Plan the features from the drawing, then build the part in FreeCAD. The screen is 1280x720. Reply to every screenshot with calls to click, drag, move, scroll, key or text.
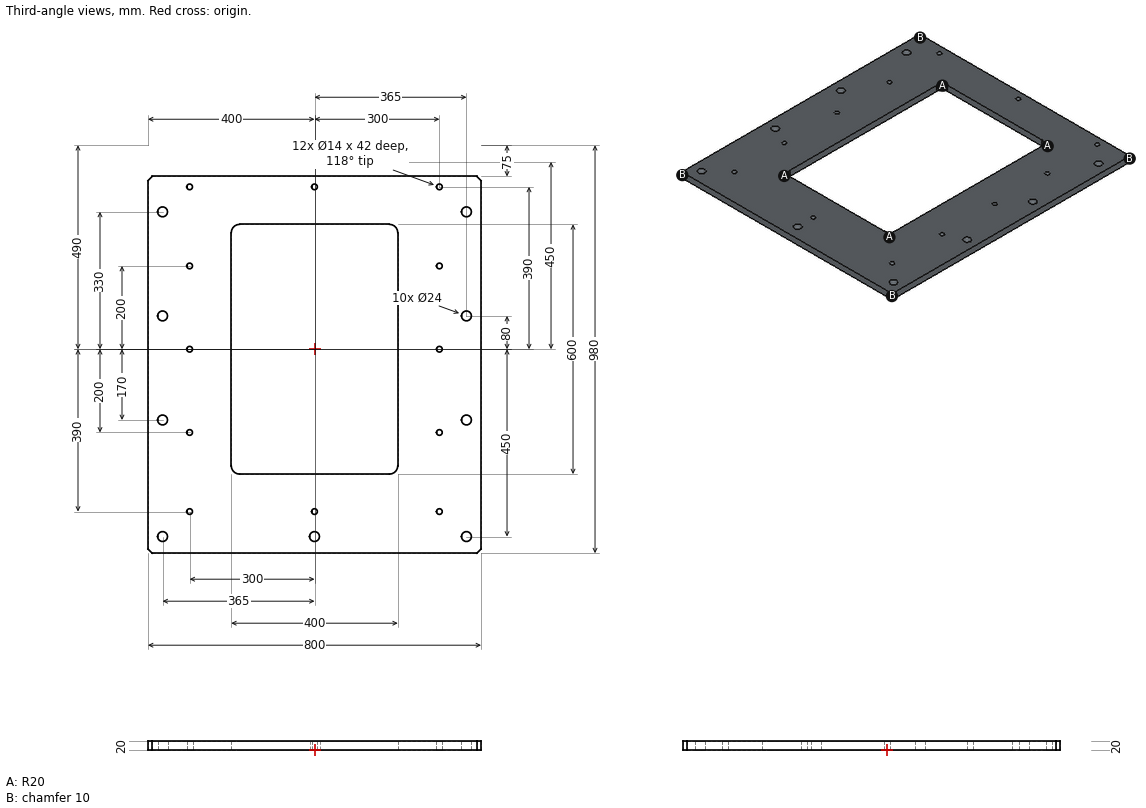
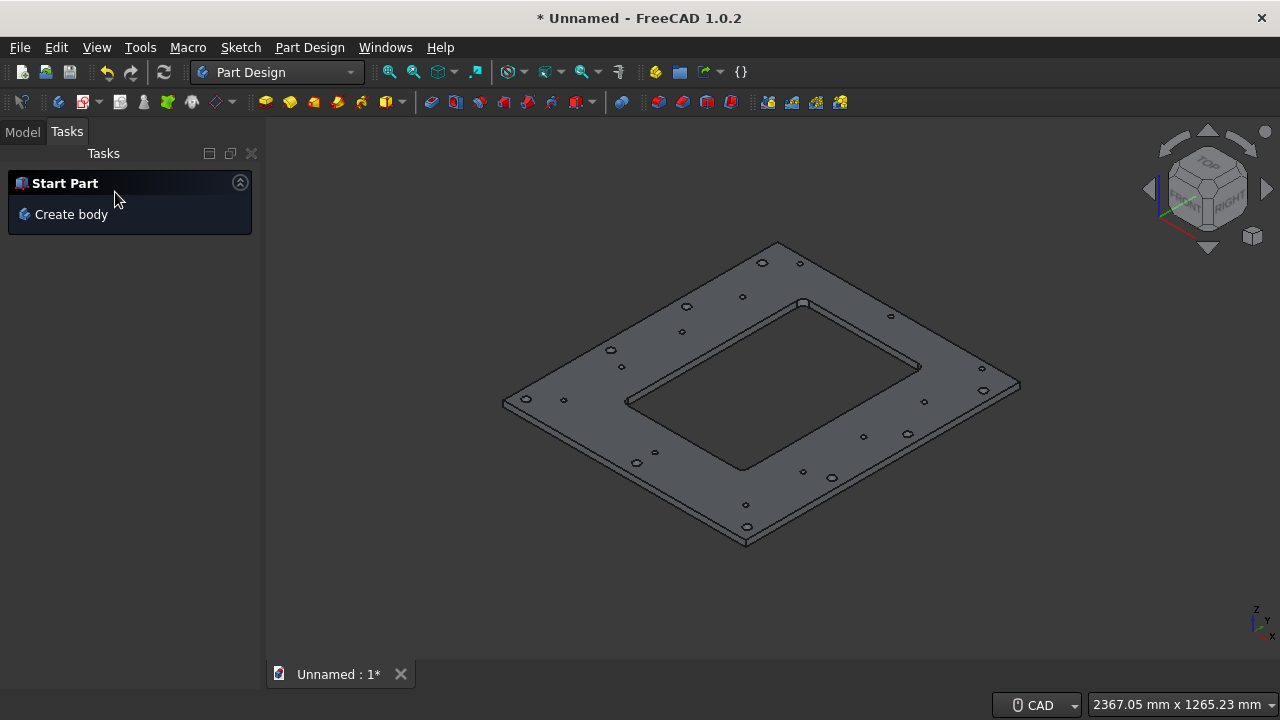
scroll(778, 244, up, 8)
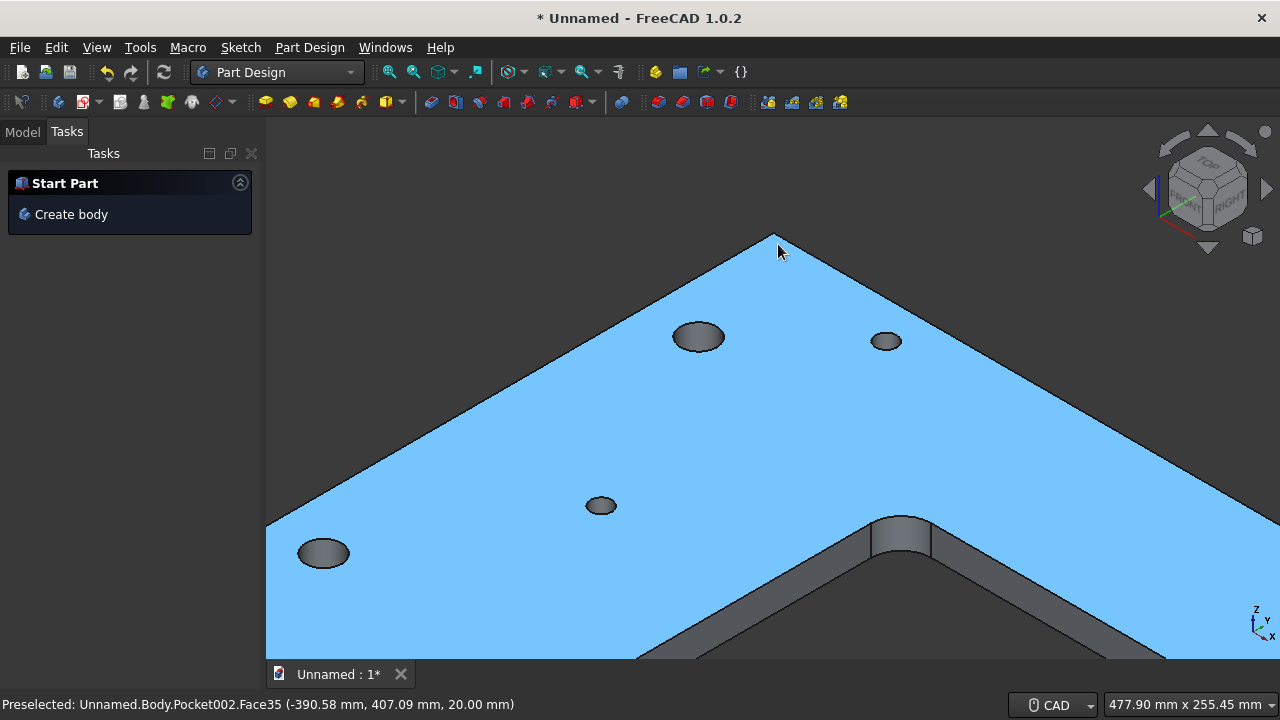
click(390, 72)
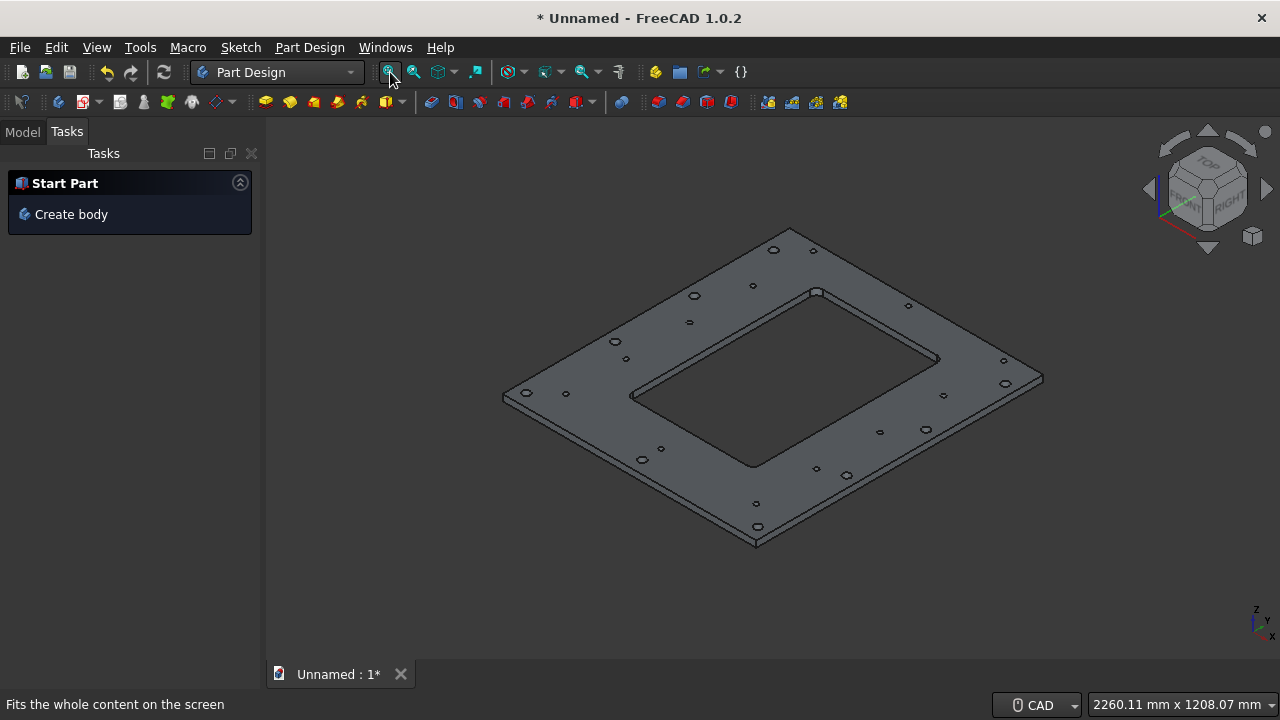
key(2)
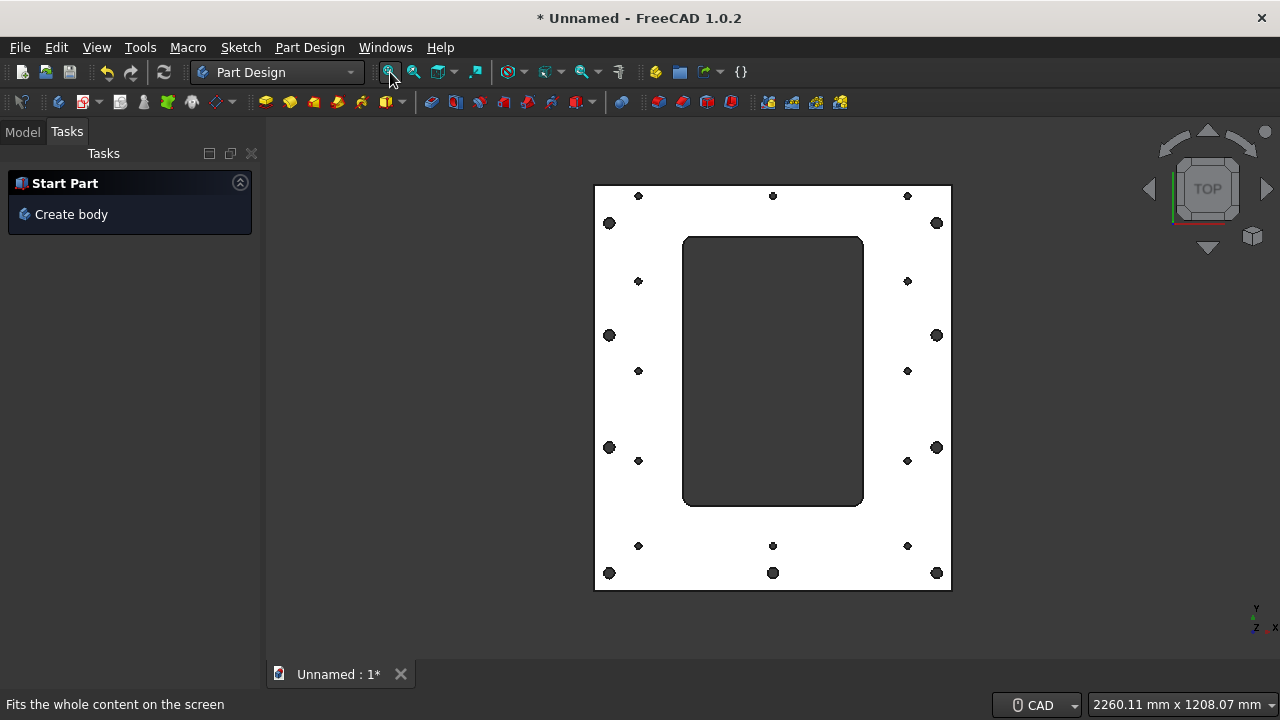
scroll(594, 184, up, 8)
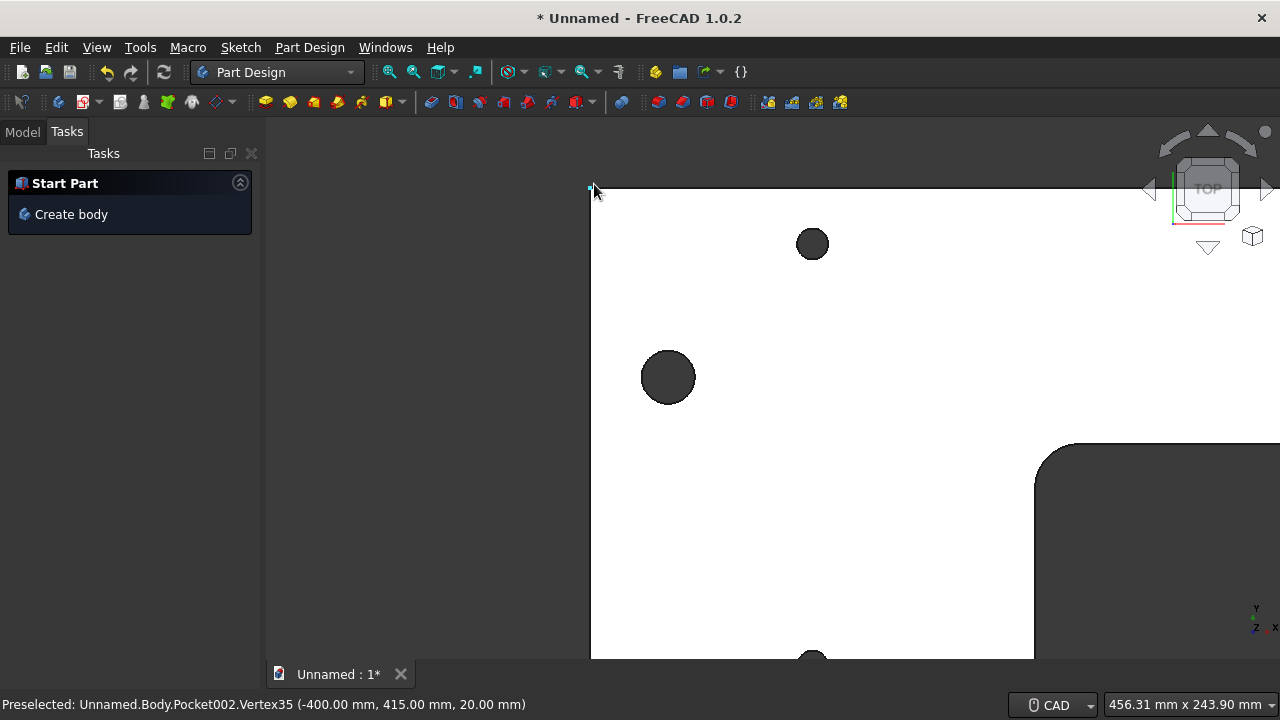
click(390, 72)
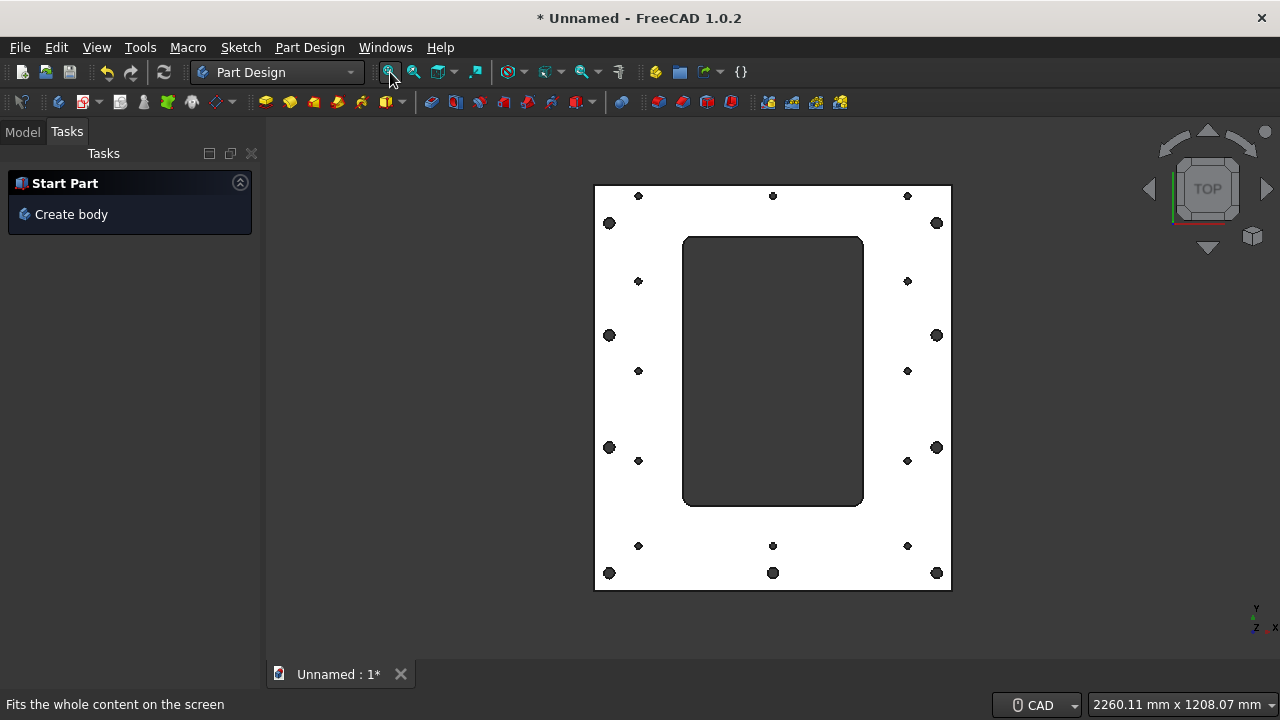
key(0)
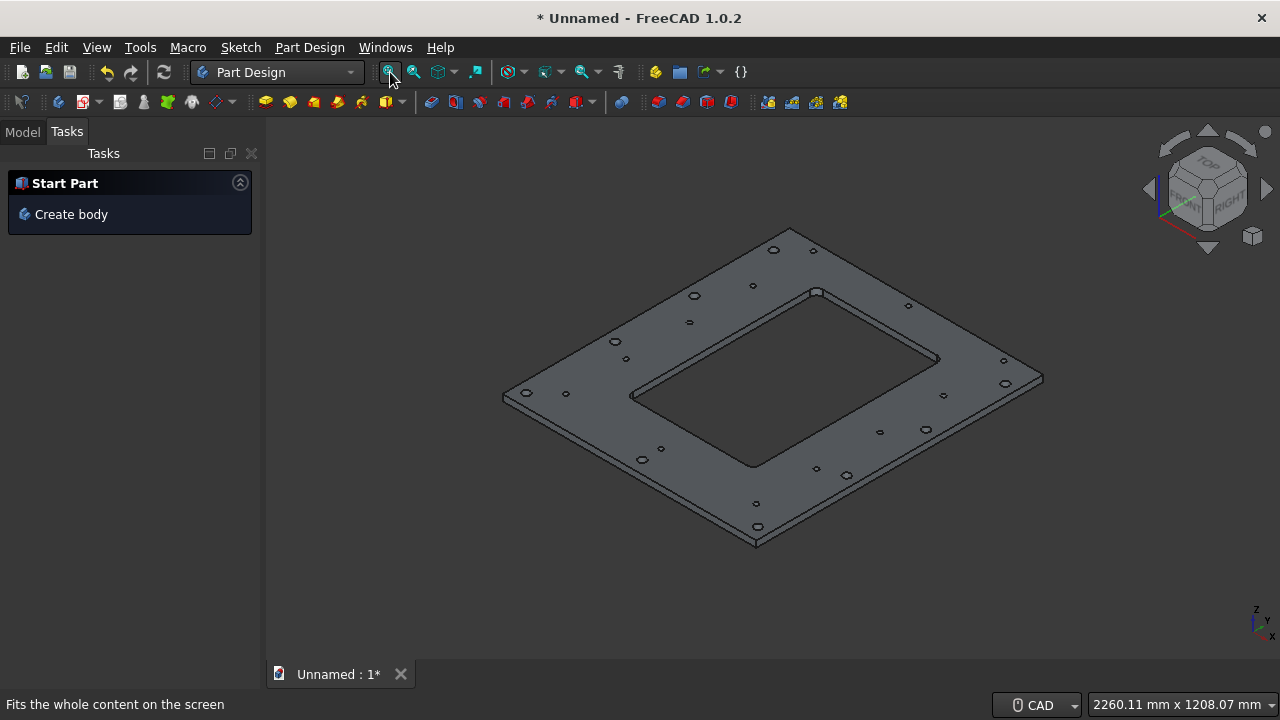
scroll(790, 231, up, 8)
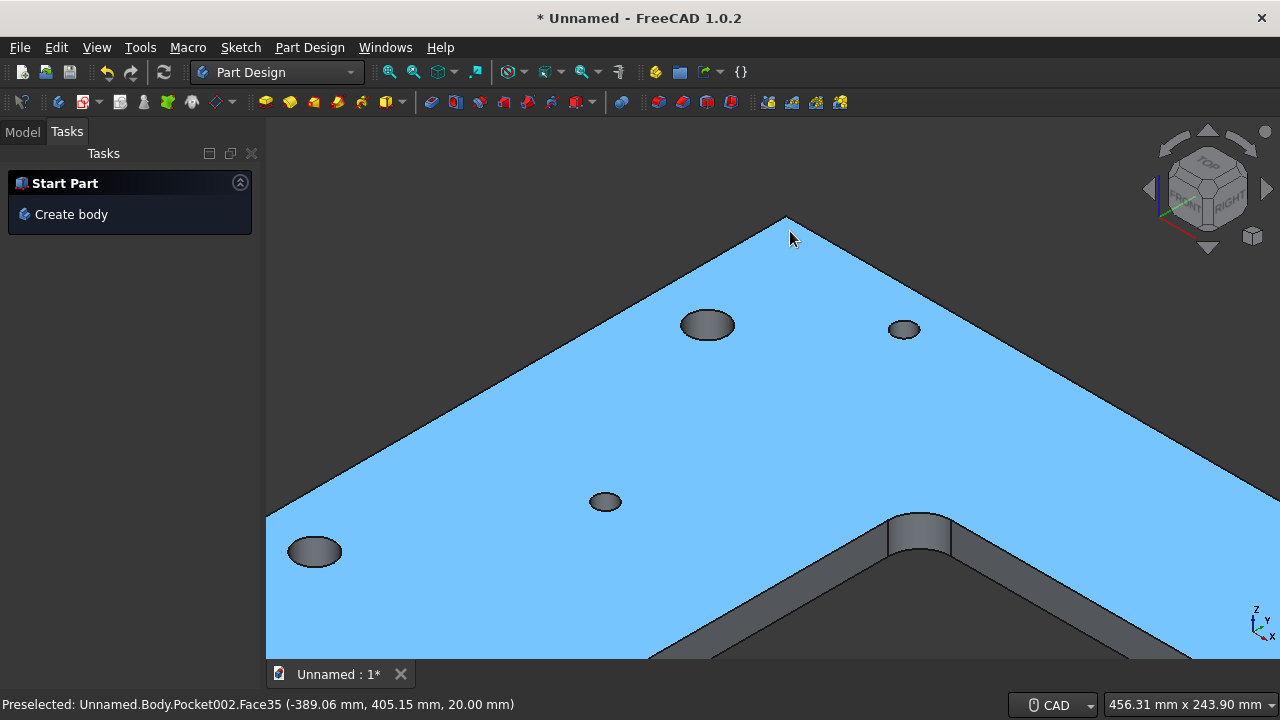
click(390, 72)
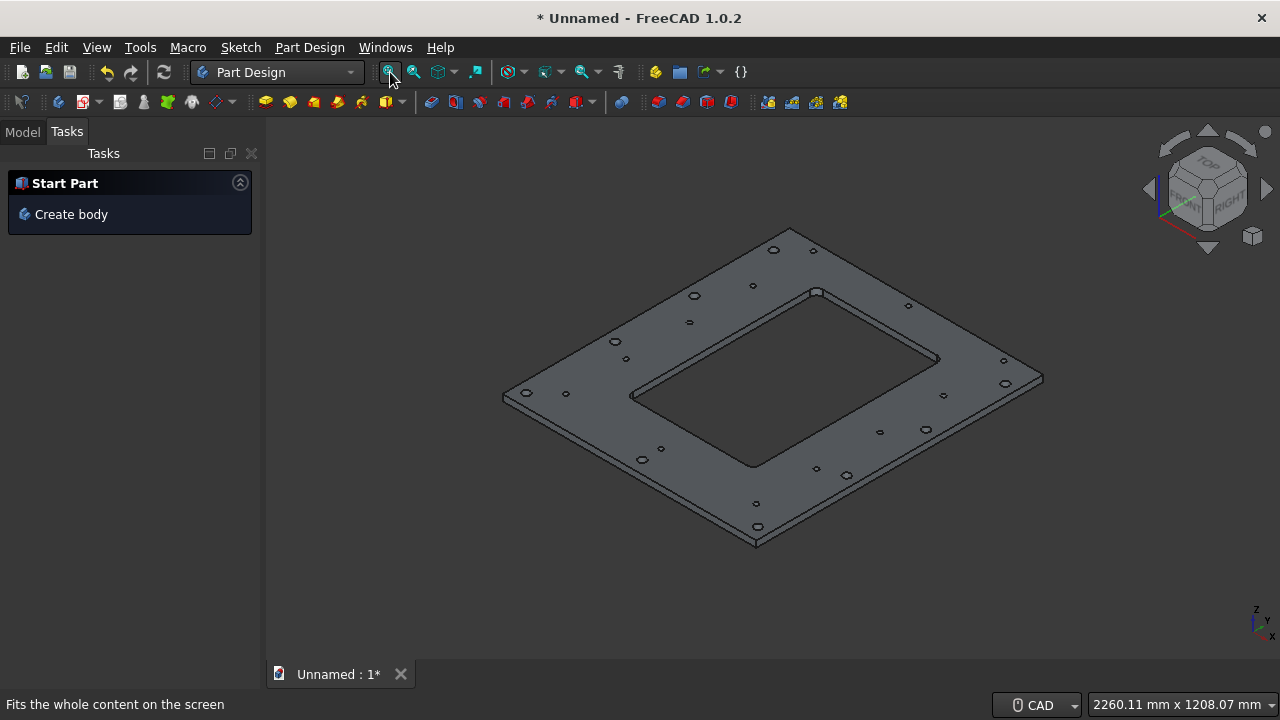
key(1)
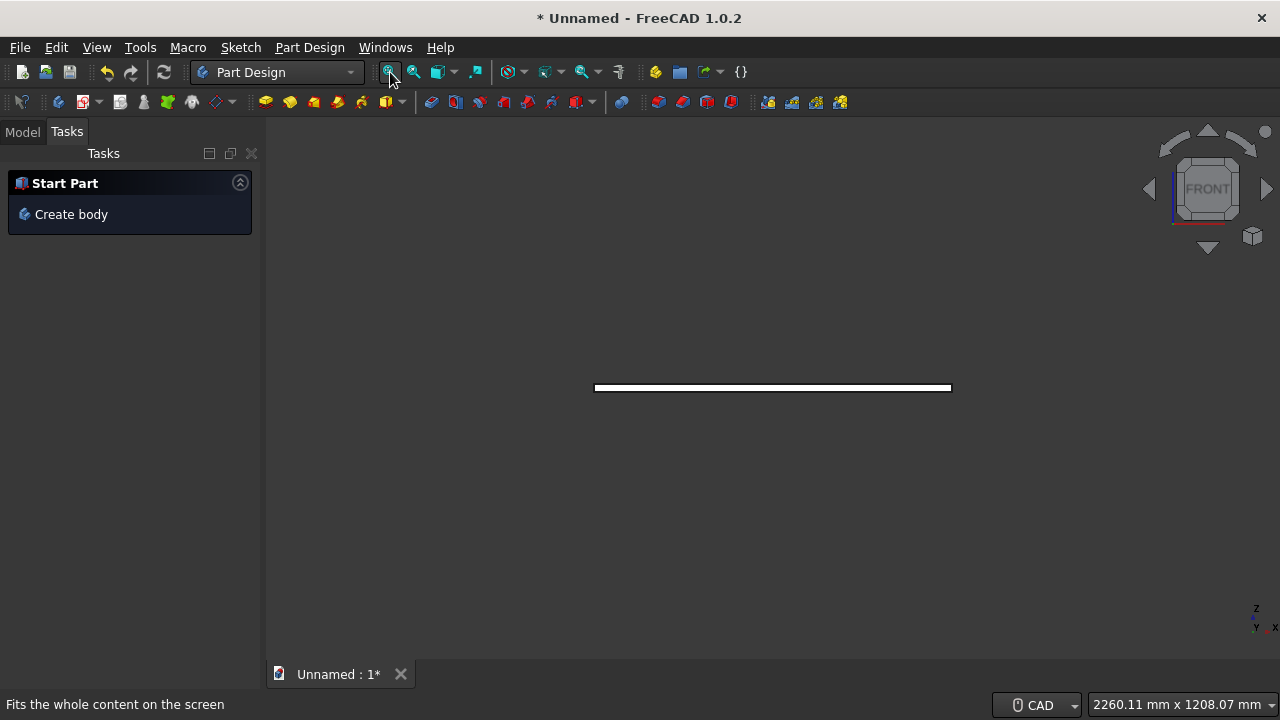
click(390, 72)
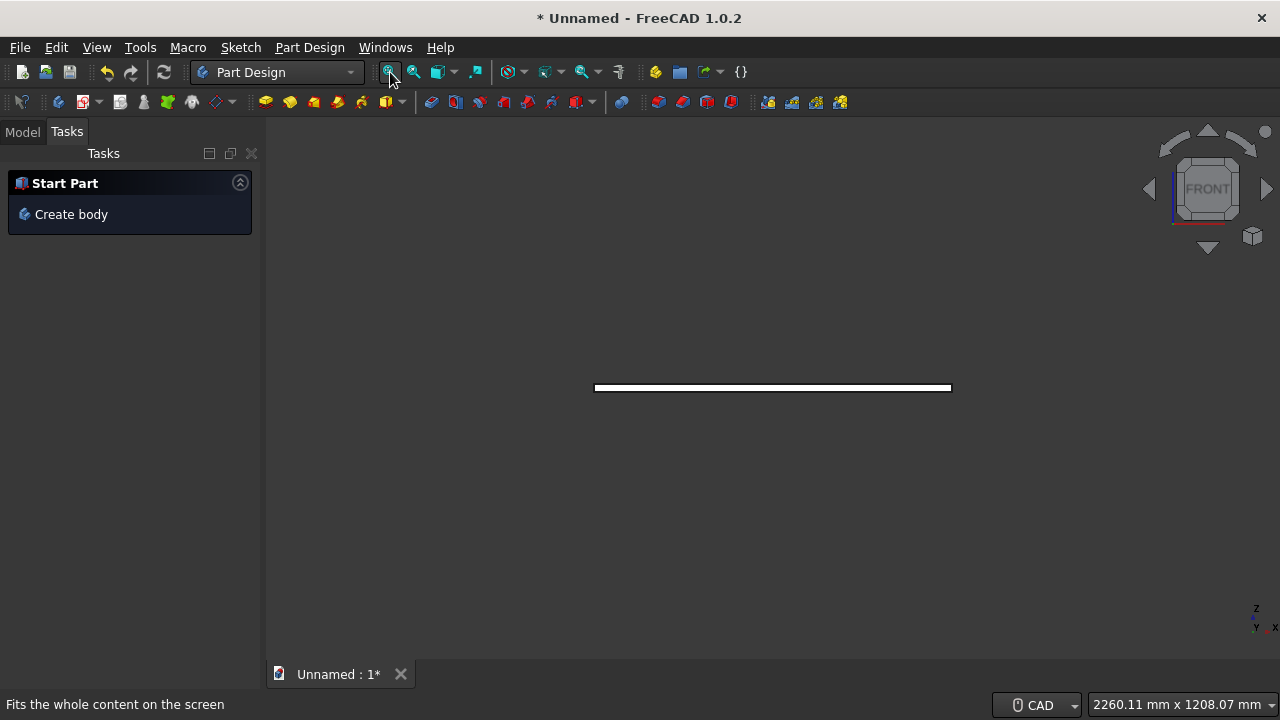
scroll(594, 387, up, 8)